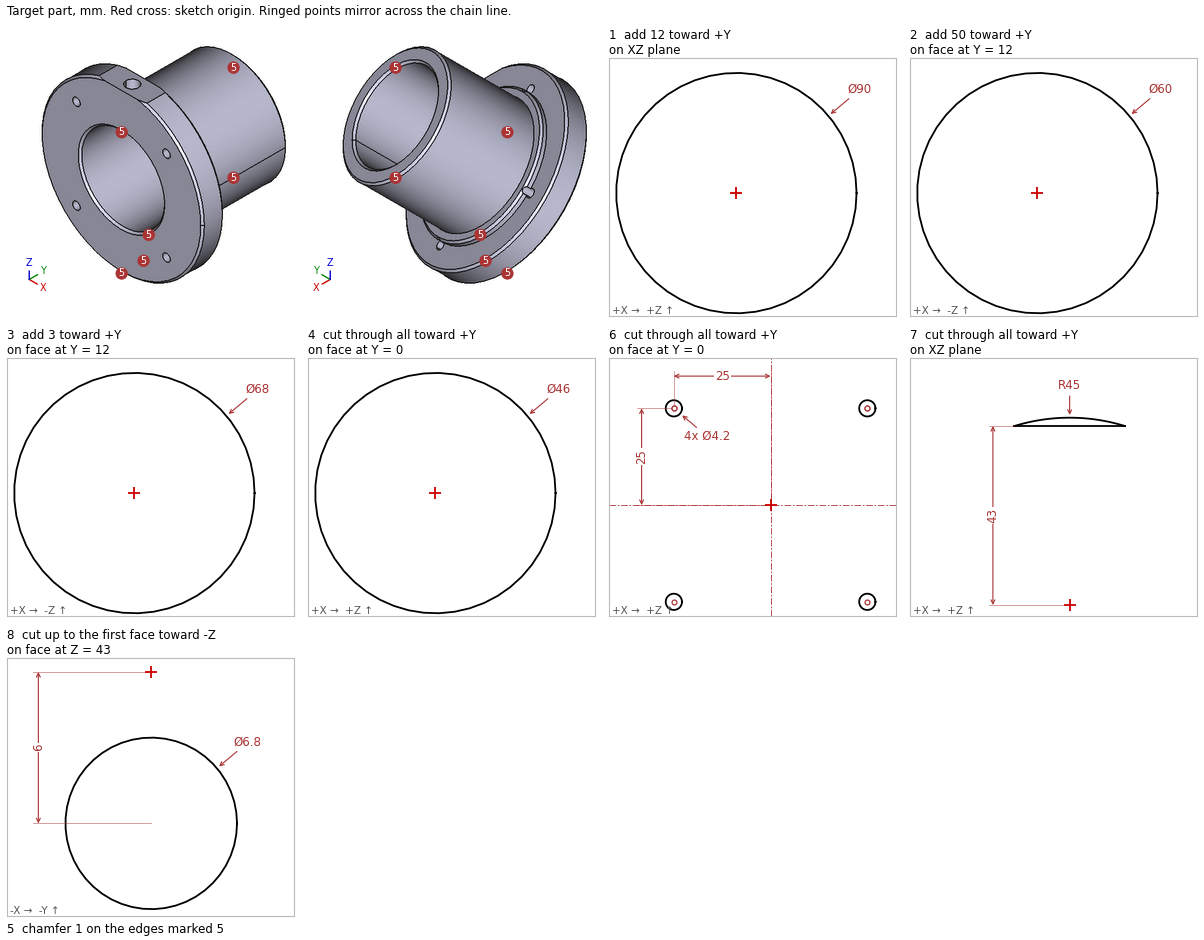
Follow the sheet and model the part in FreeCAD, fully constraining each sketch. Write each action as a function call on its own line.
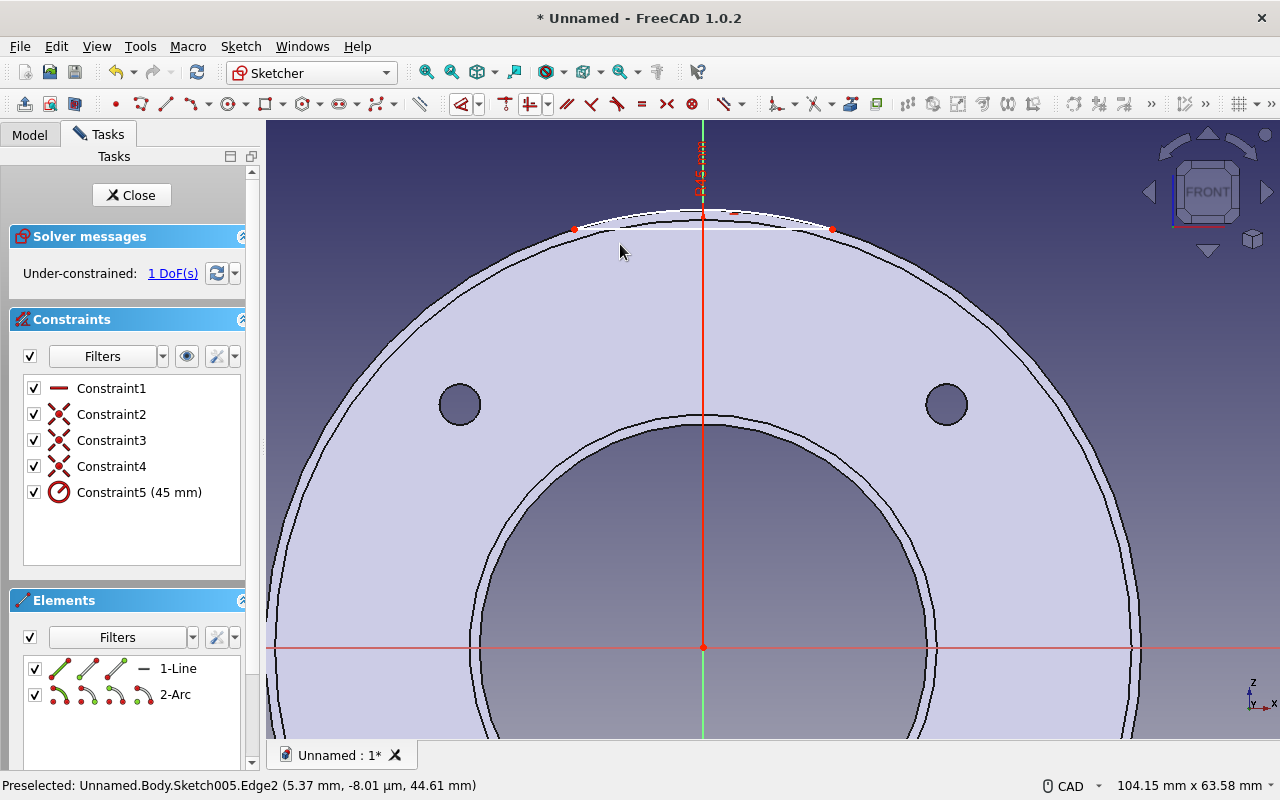
click(574, 229)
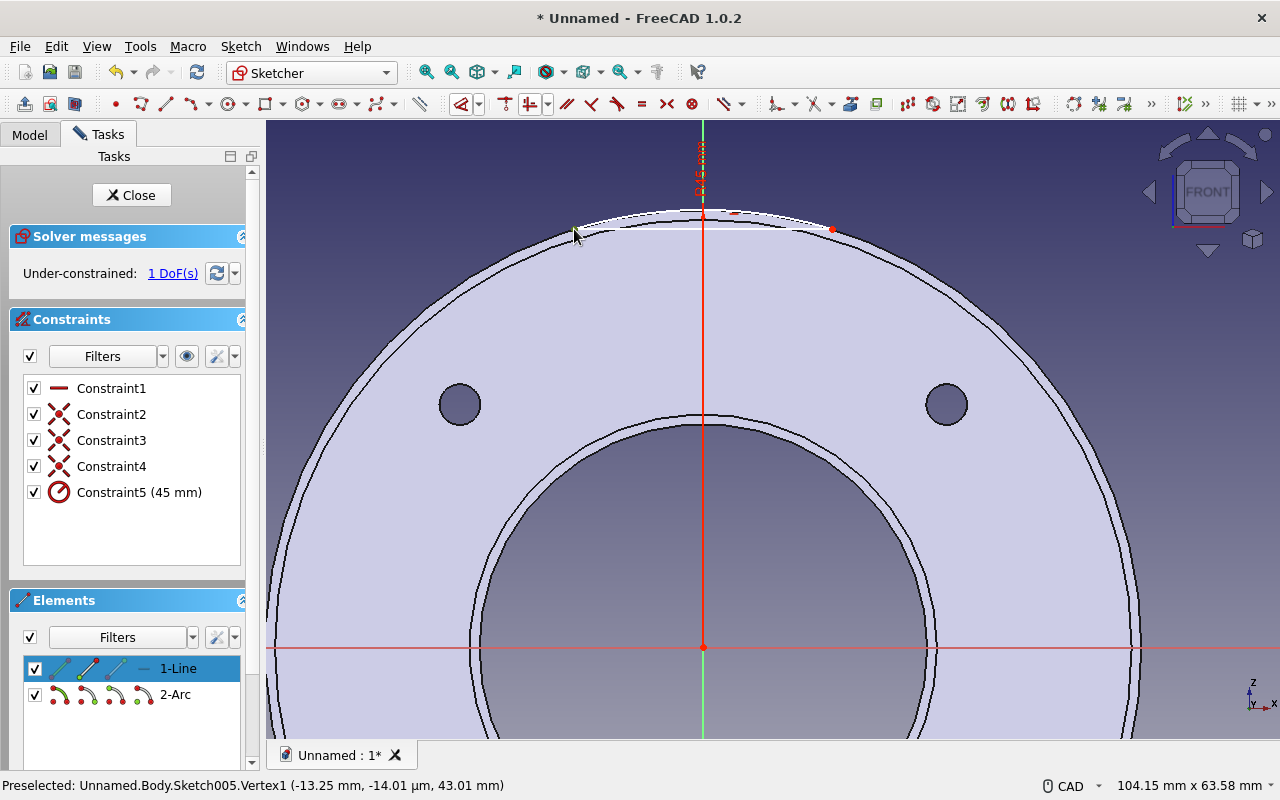
key(i)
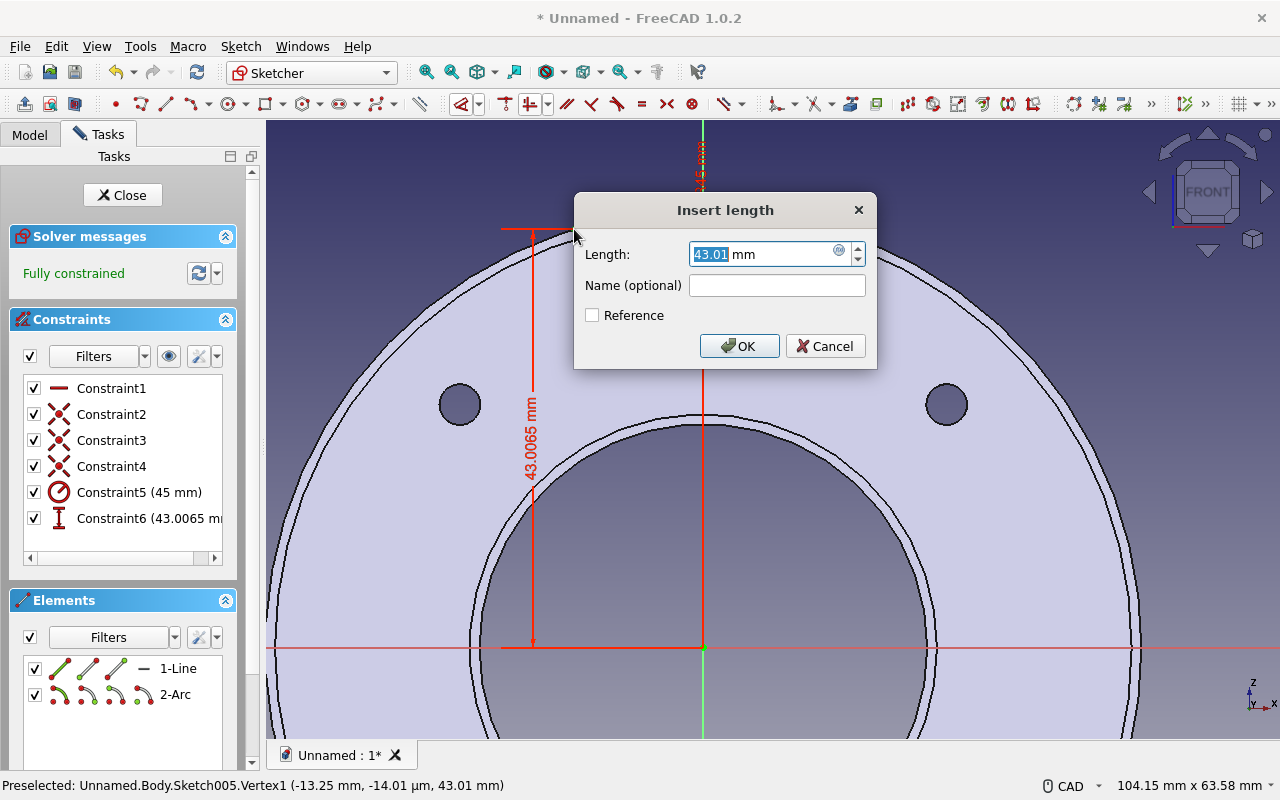
text(43)
key(Return)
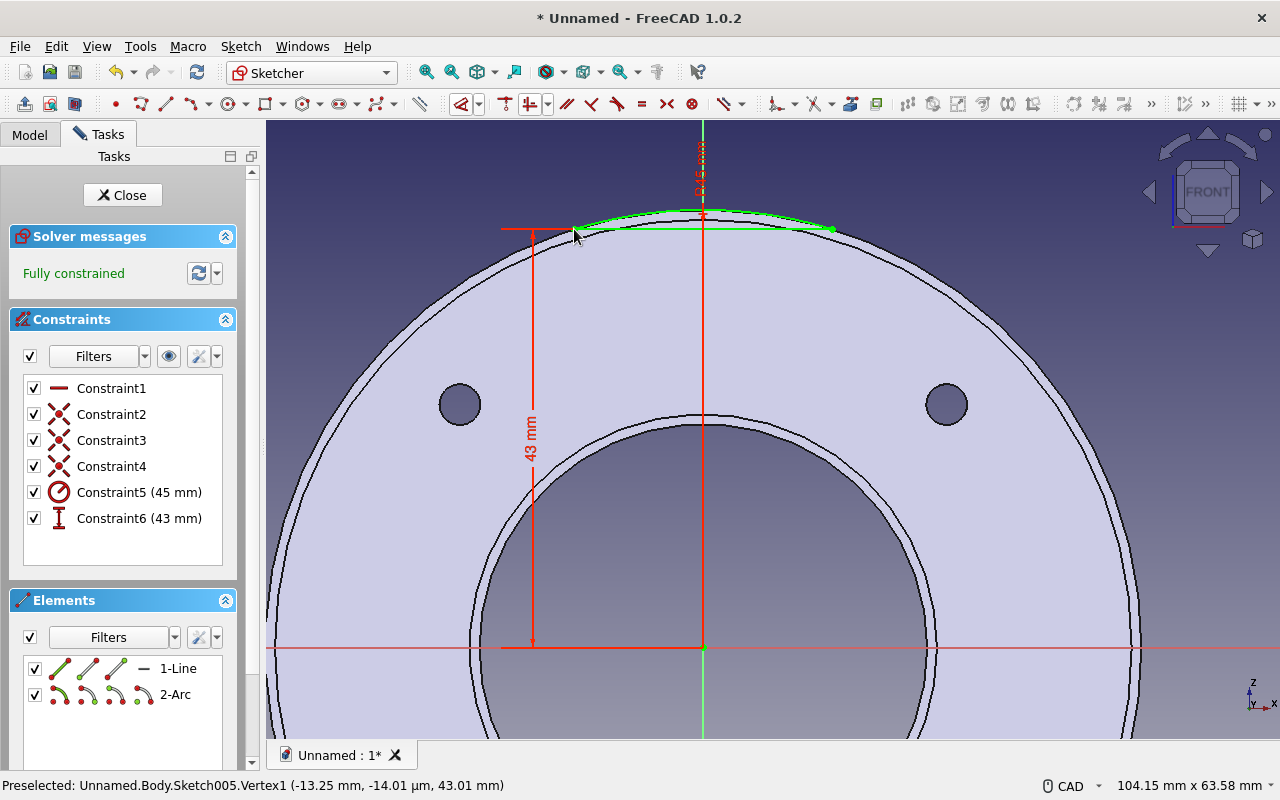
click(123, 195)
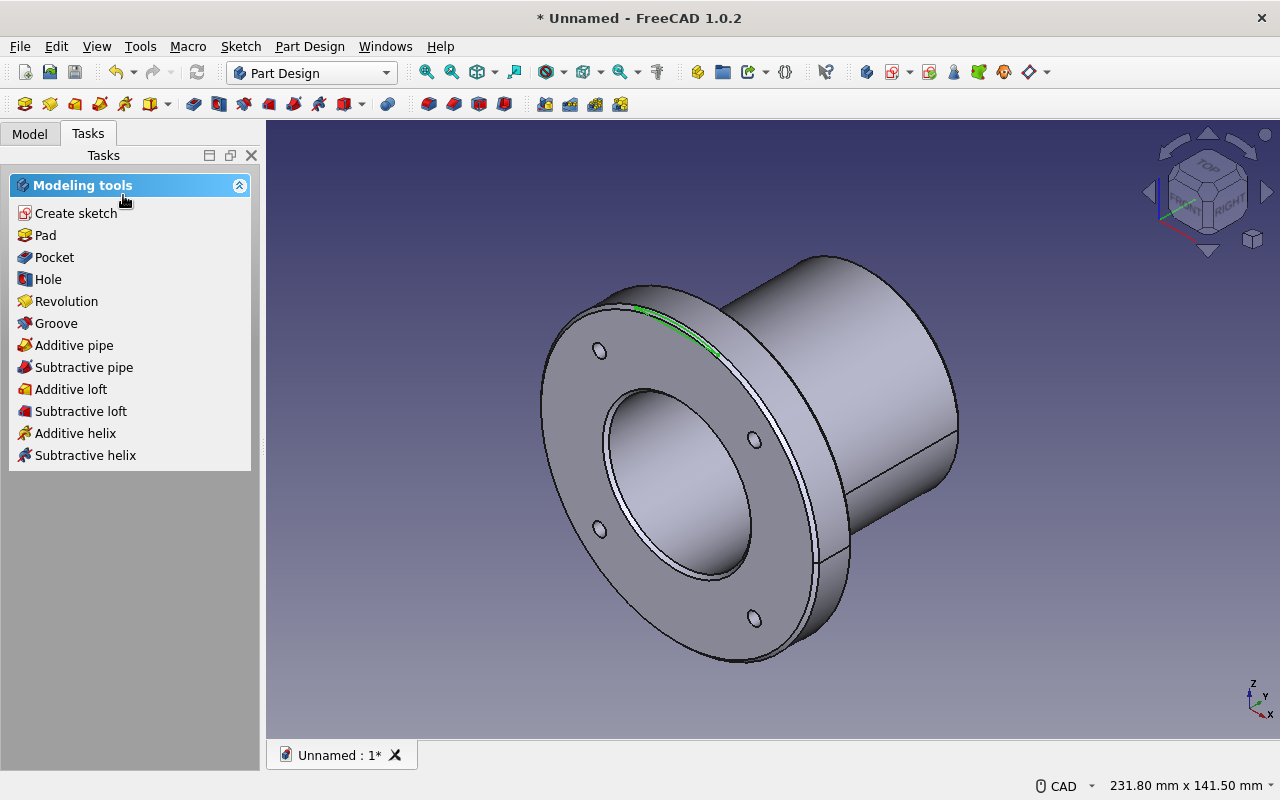
click(194, 104)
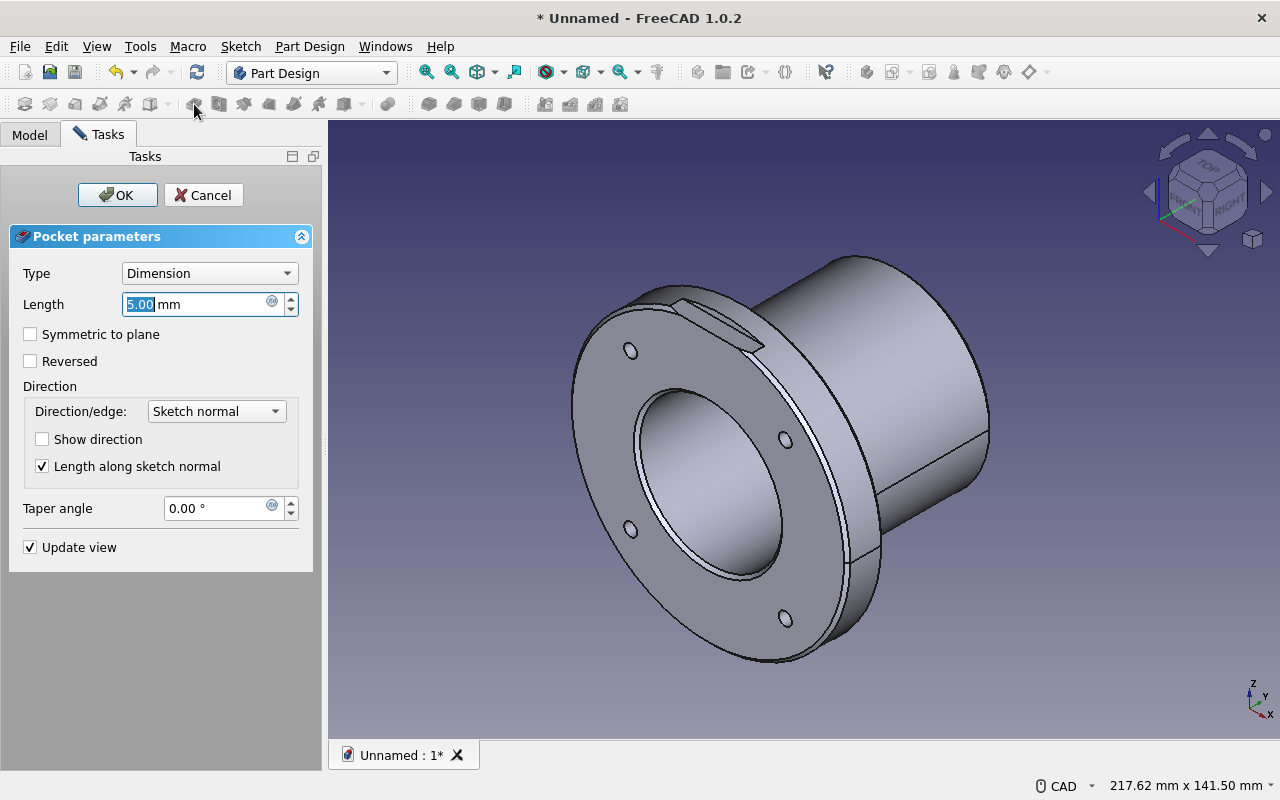
click(210, 274)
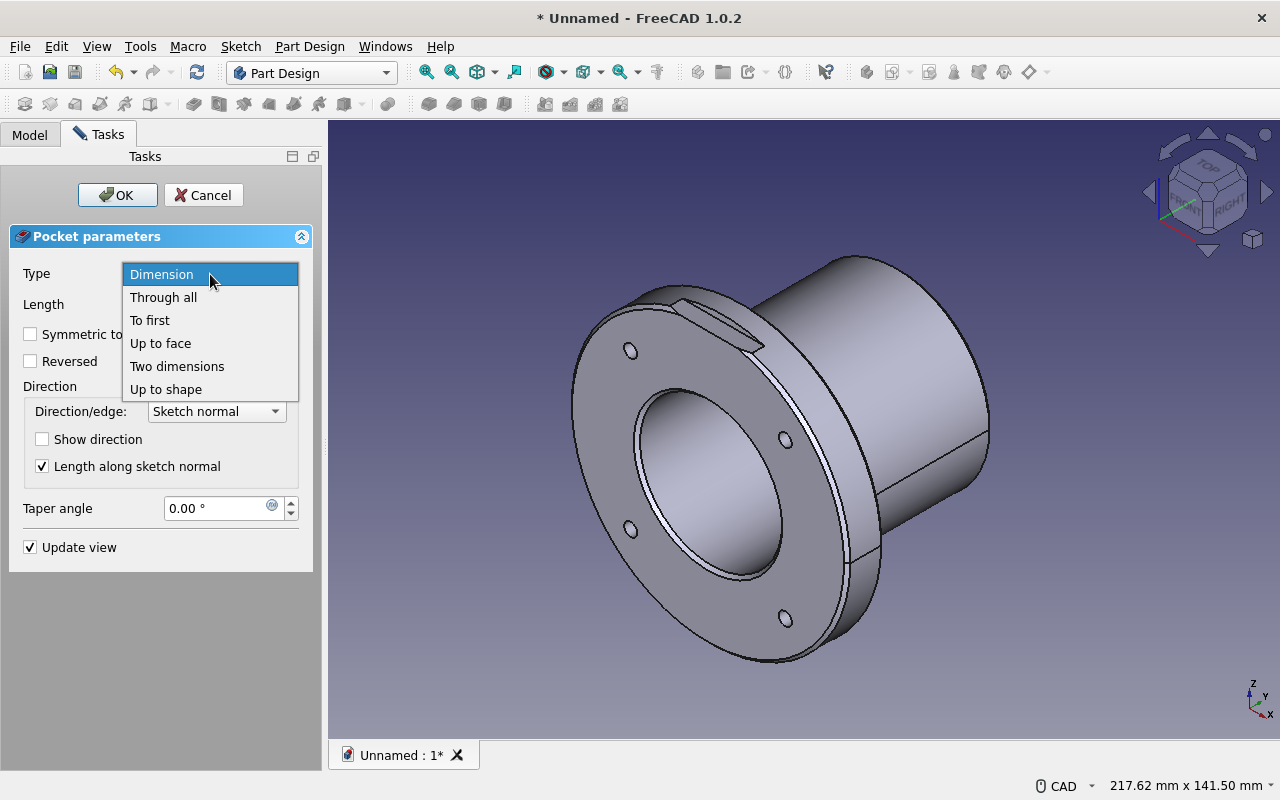
click(208, 298)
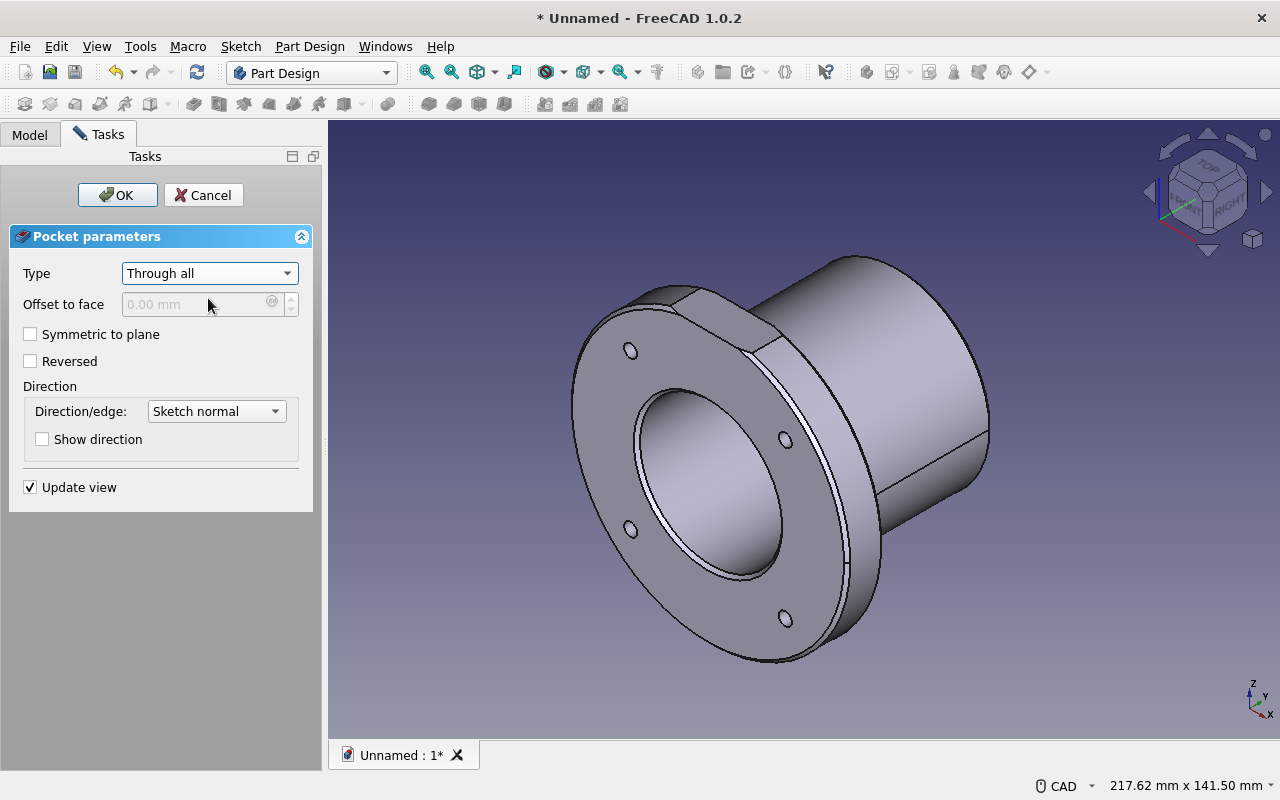
click(118, 195)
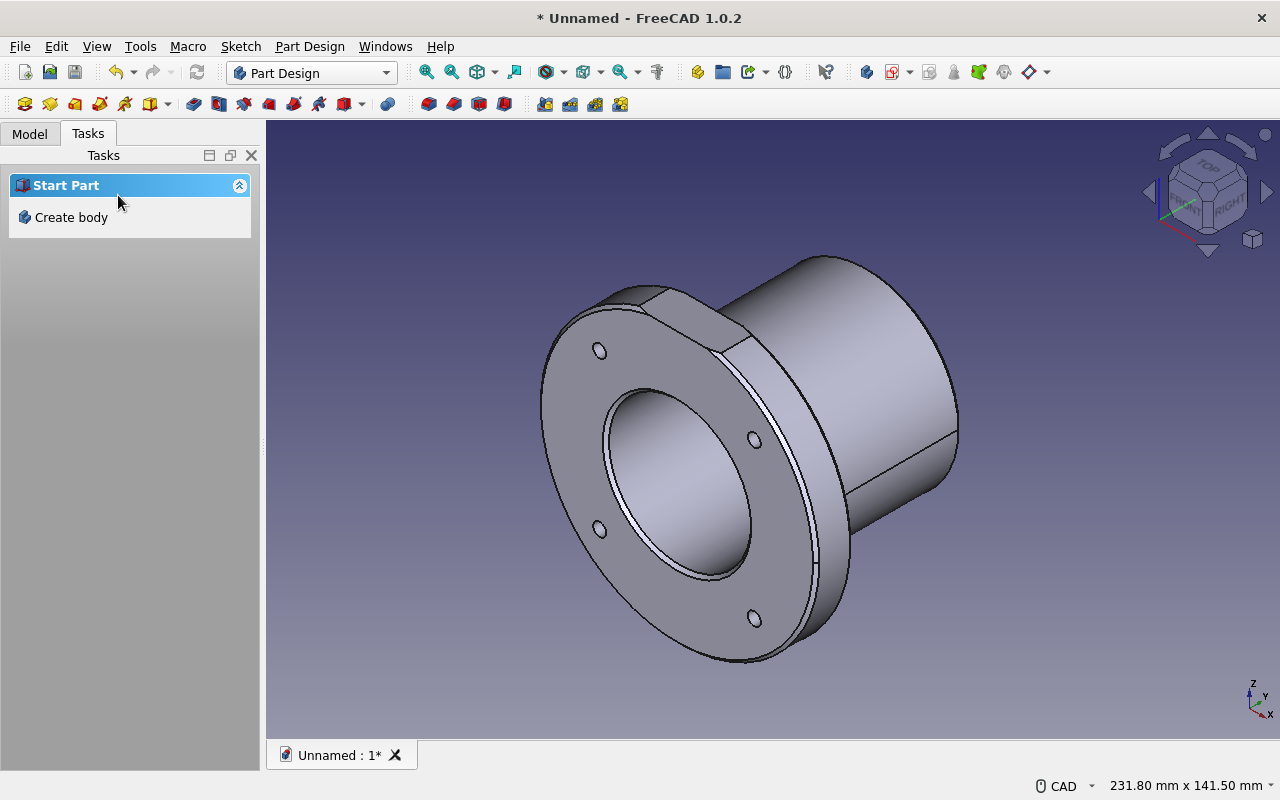
click(707, 326)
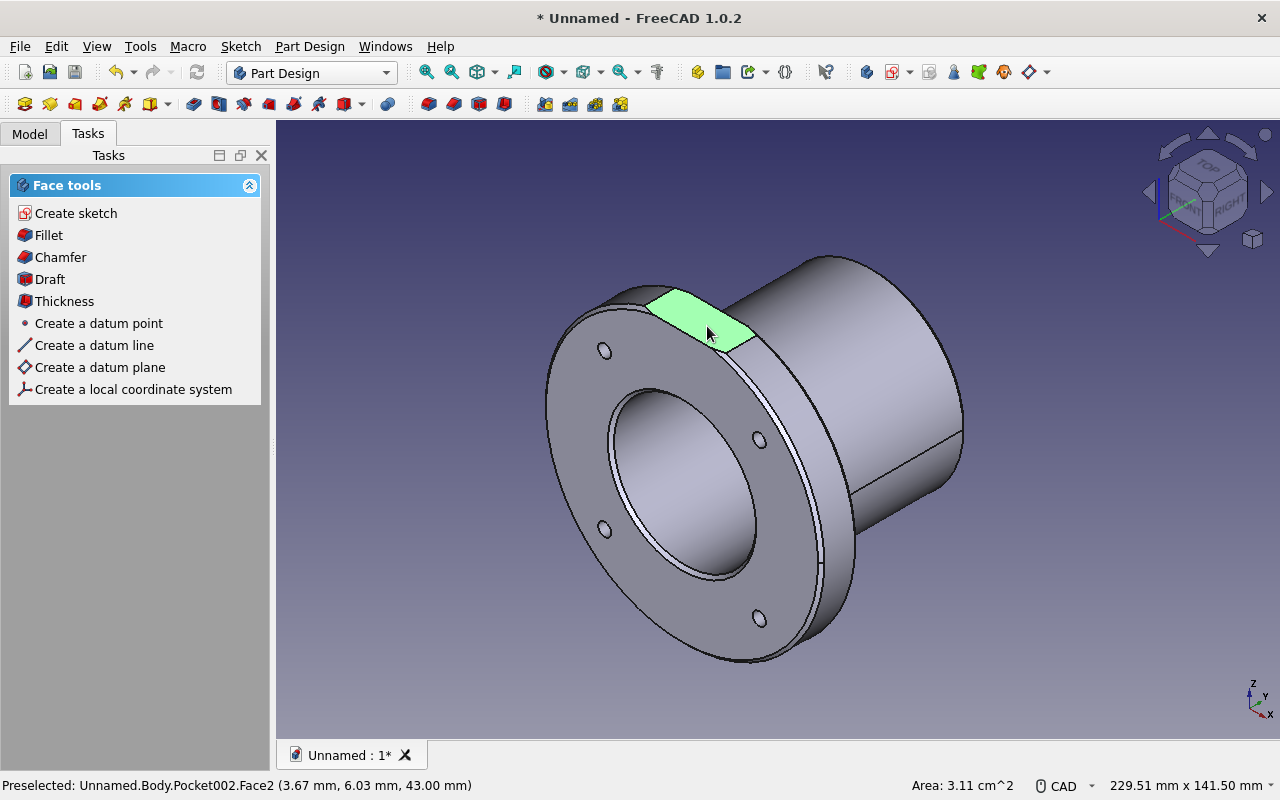
click(892, 72)